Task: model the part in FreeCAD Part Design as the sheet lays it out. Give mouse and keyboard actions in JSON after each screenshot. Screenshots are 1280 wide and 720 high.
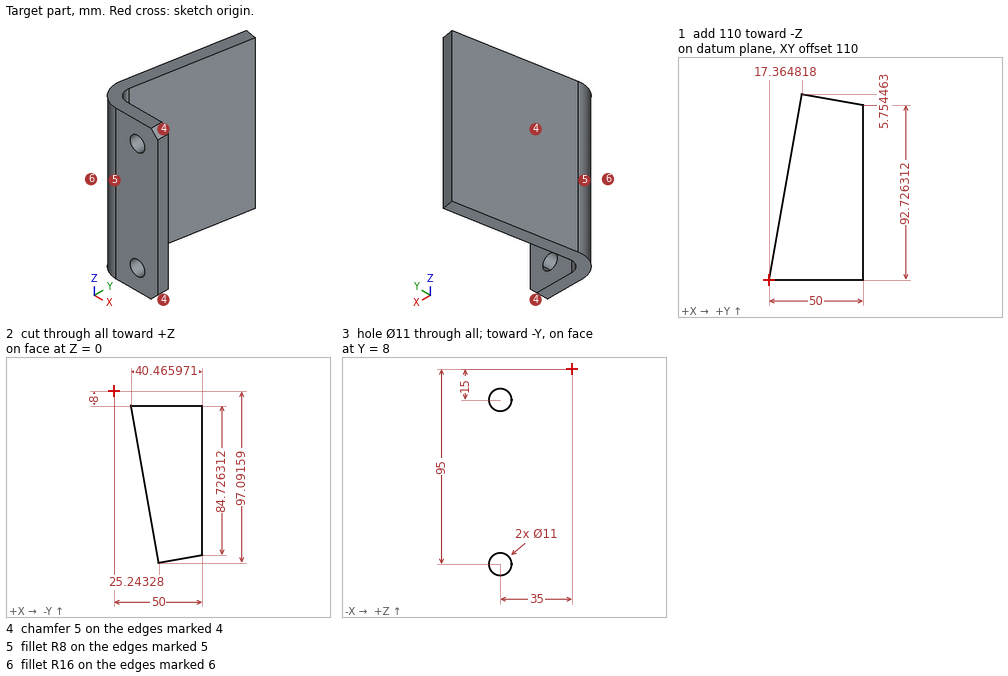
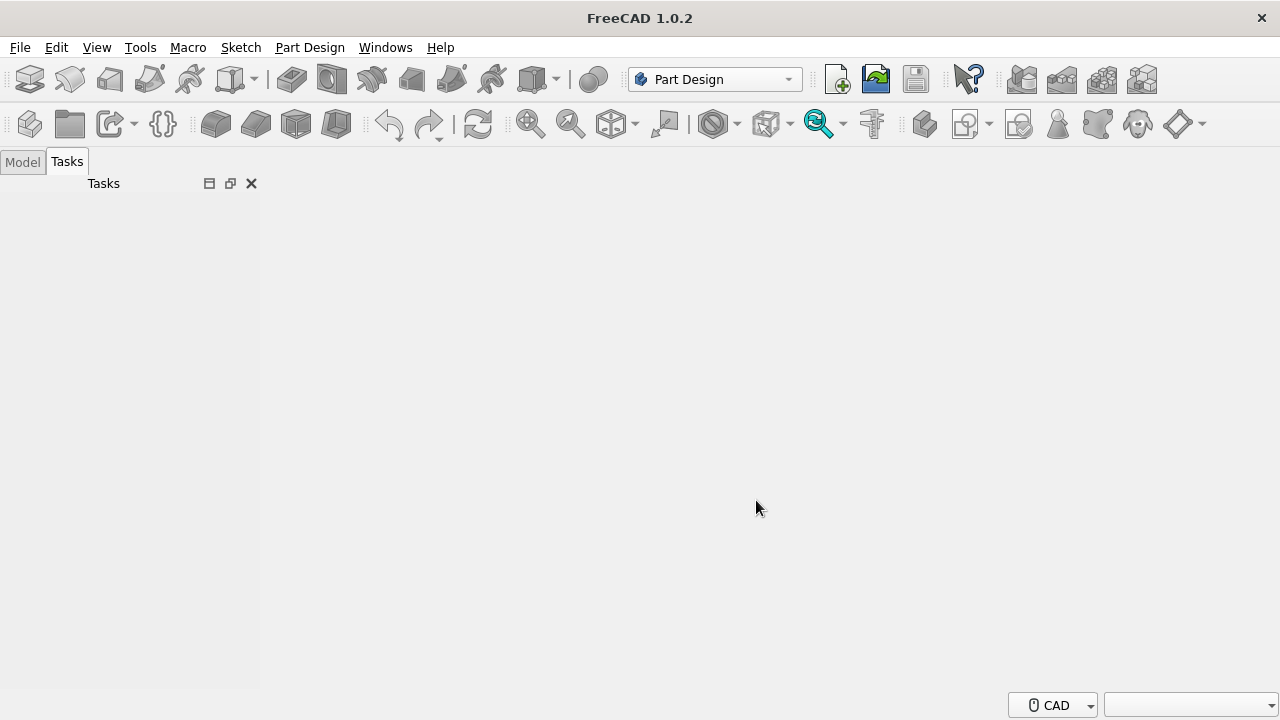
{"action": "left_click", "coordinate": [836, 80]}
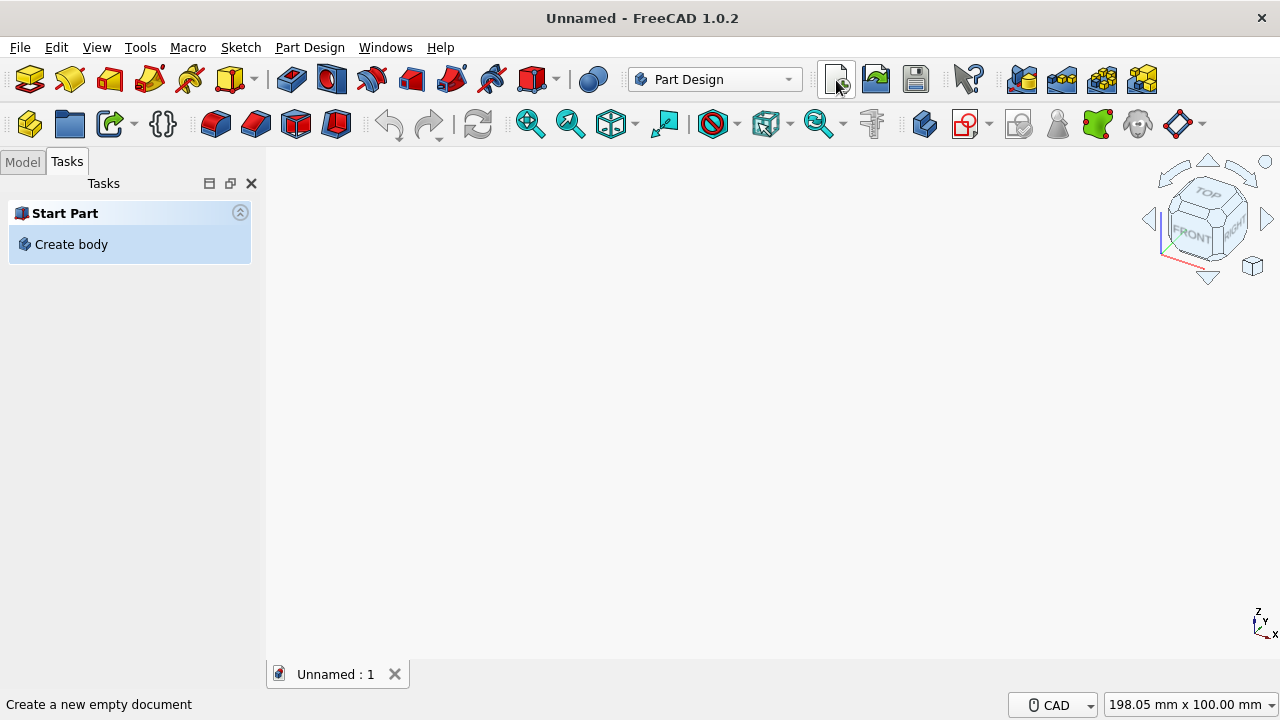
{"action": "left_click", "coordinate": [926, 124]}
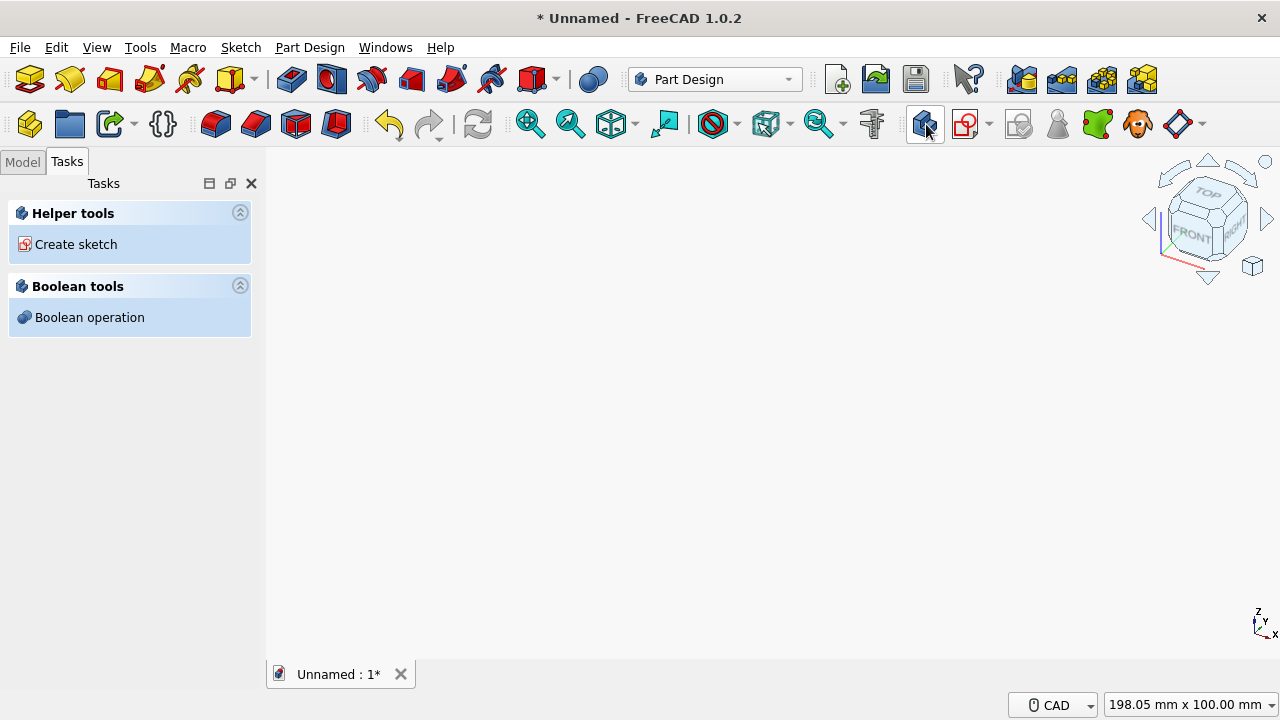
{"action": "left_click", "coordinate": [23, 161]}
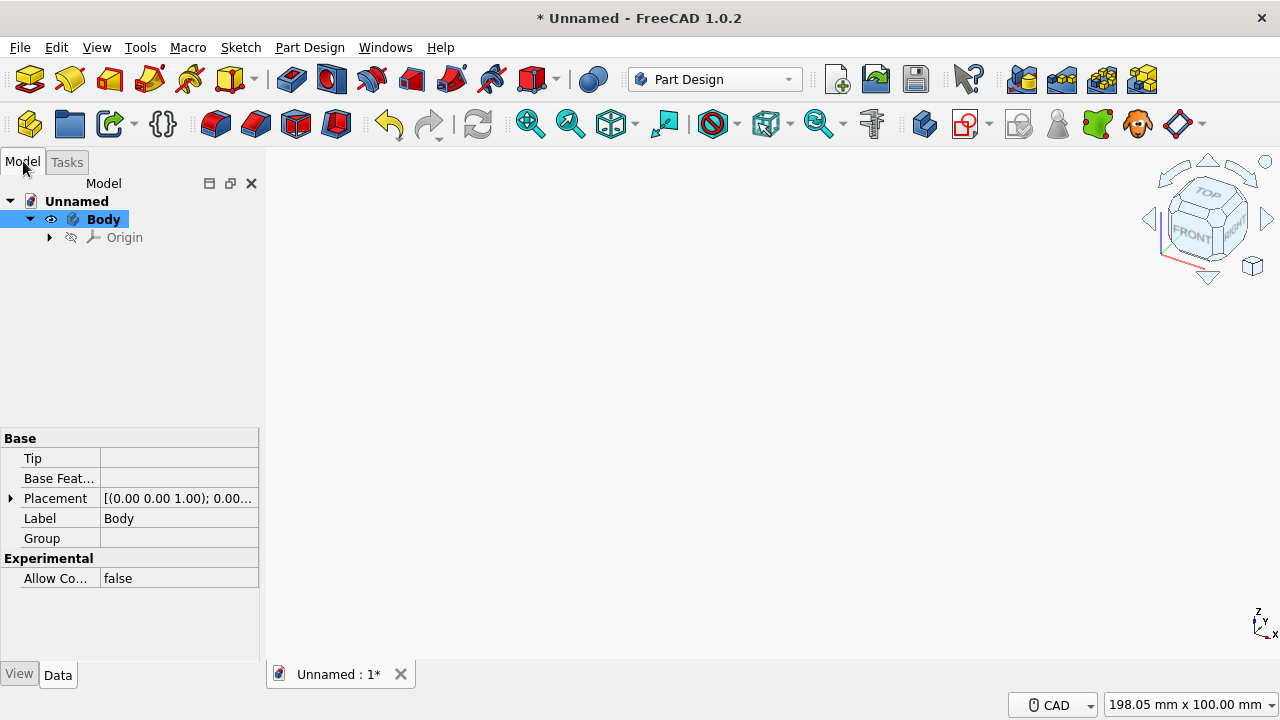
{"action": "left_click", "coordinate": [50, 237]}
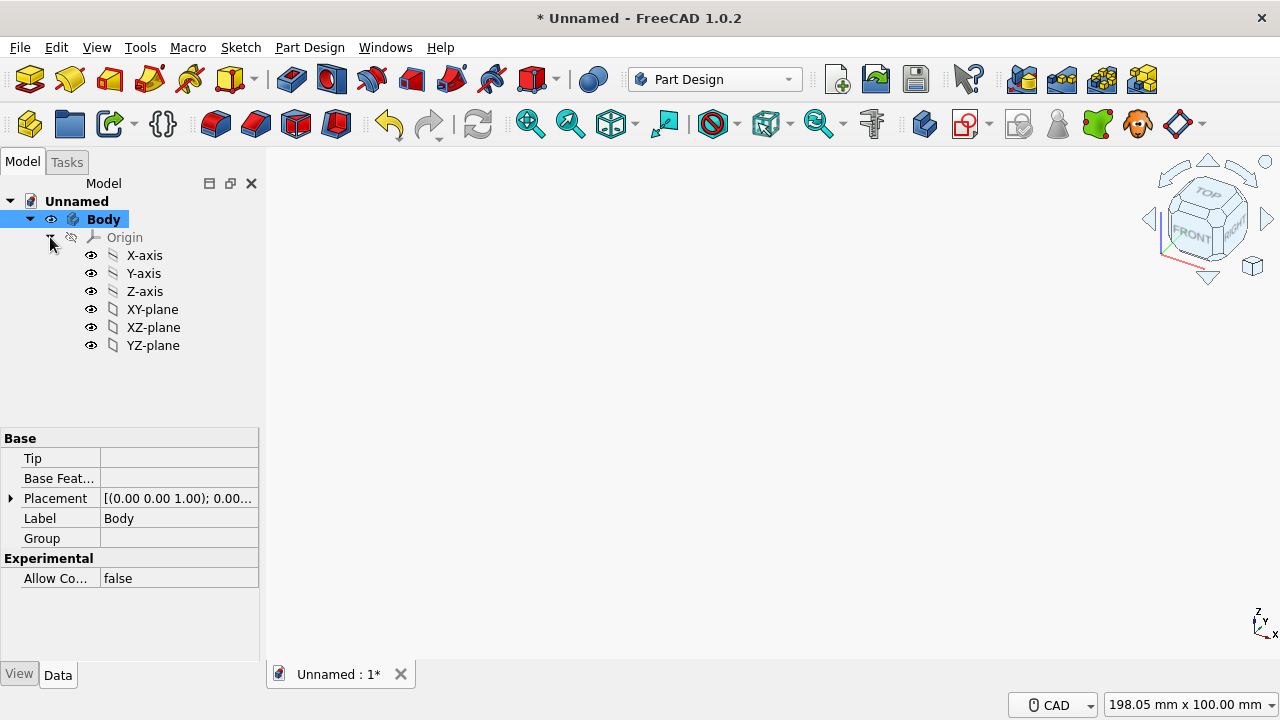
{"action": "left_click", "coordinate": [136, 309]}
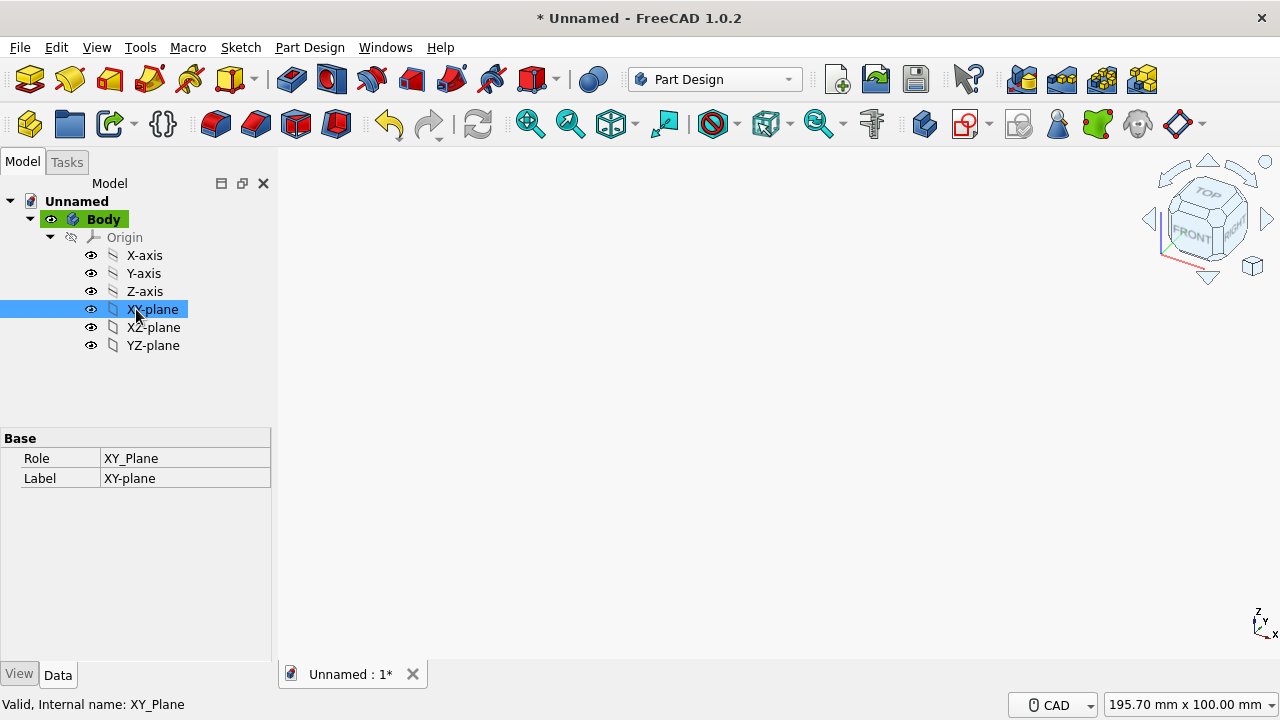
{"action": "left_click", "coordinate": [1178, 124]}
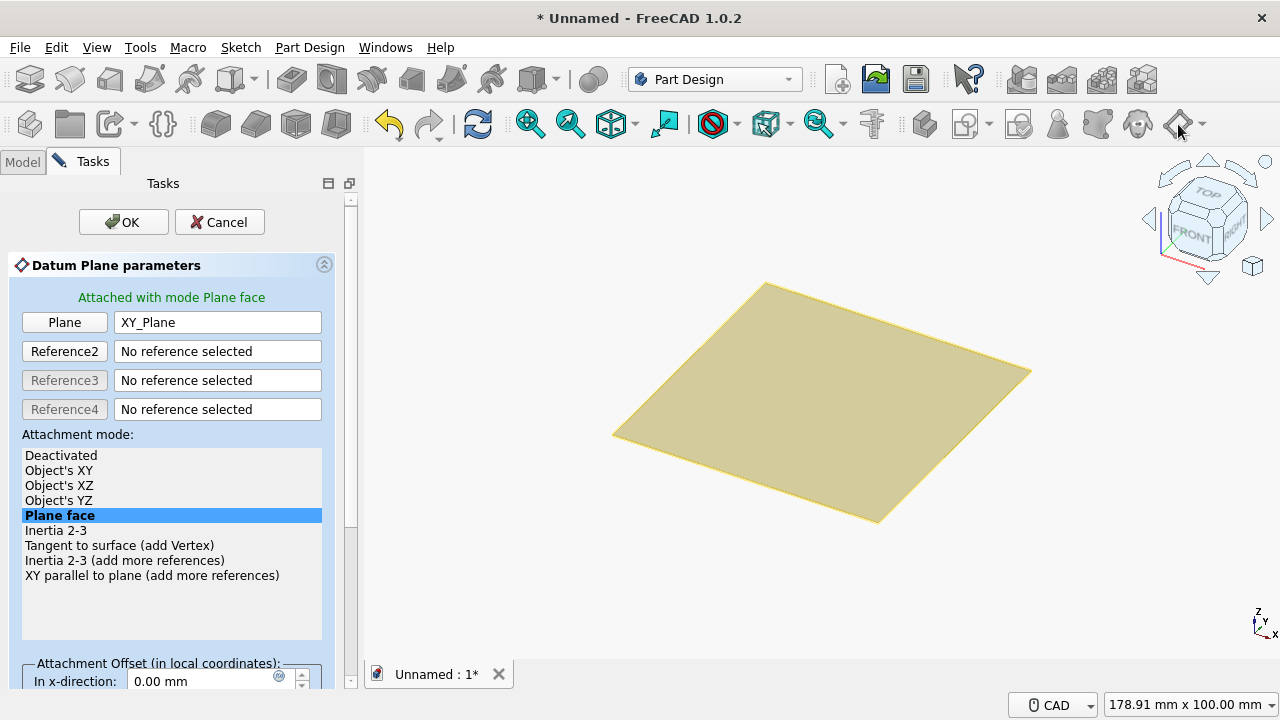
{"action": "scroll", "coordinate": [351, 440], "scroll_direction": "down", "scroll_amount": 3}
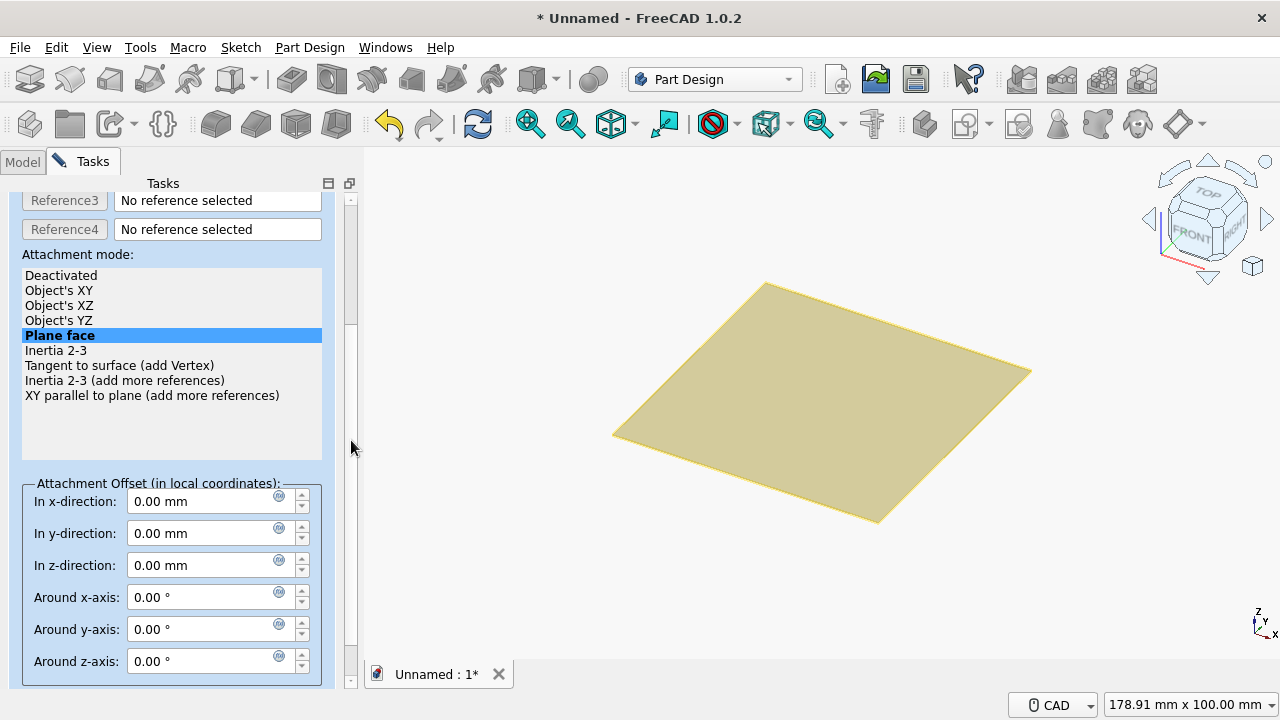
{"action": "triple_click", "coordinate": [210, 565]}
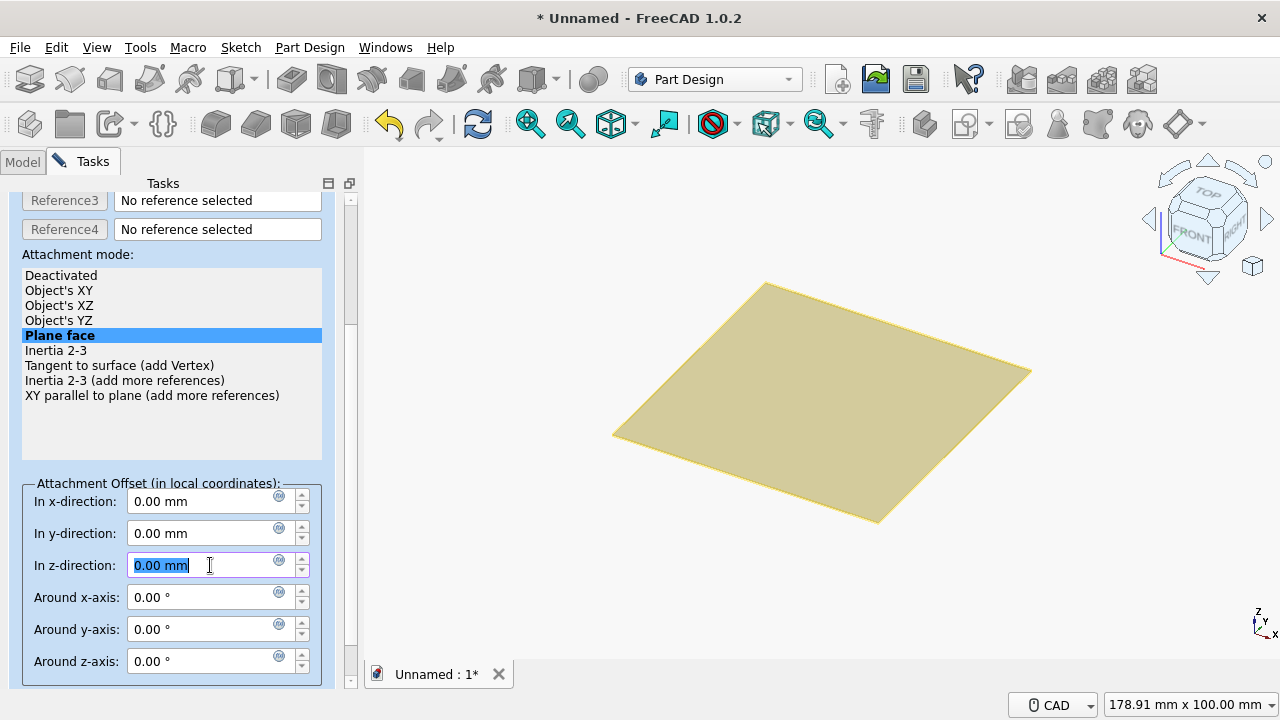
{"action": "type", "text": "110"}
{"action": "key", "text": "Tab"}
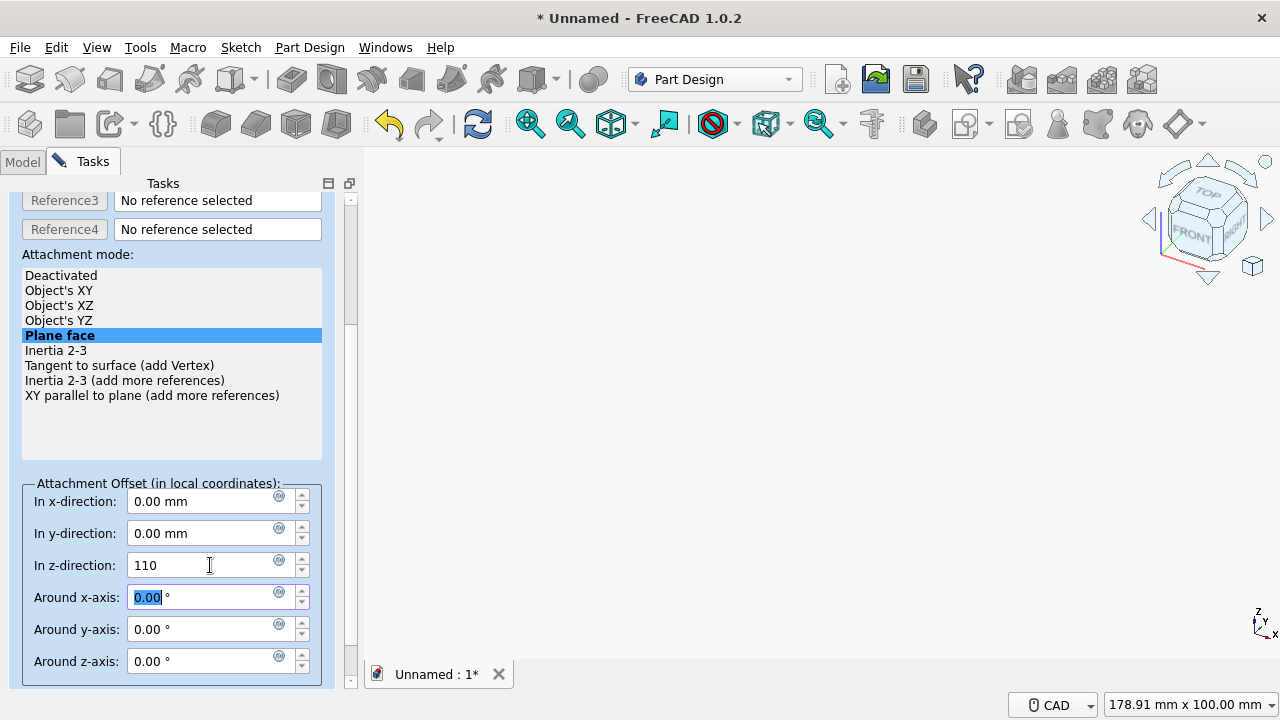
{"action": "scroll", "coordinate": [351, 440], "scroll_direction": "up", "scroll_amount": 4}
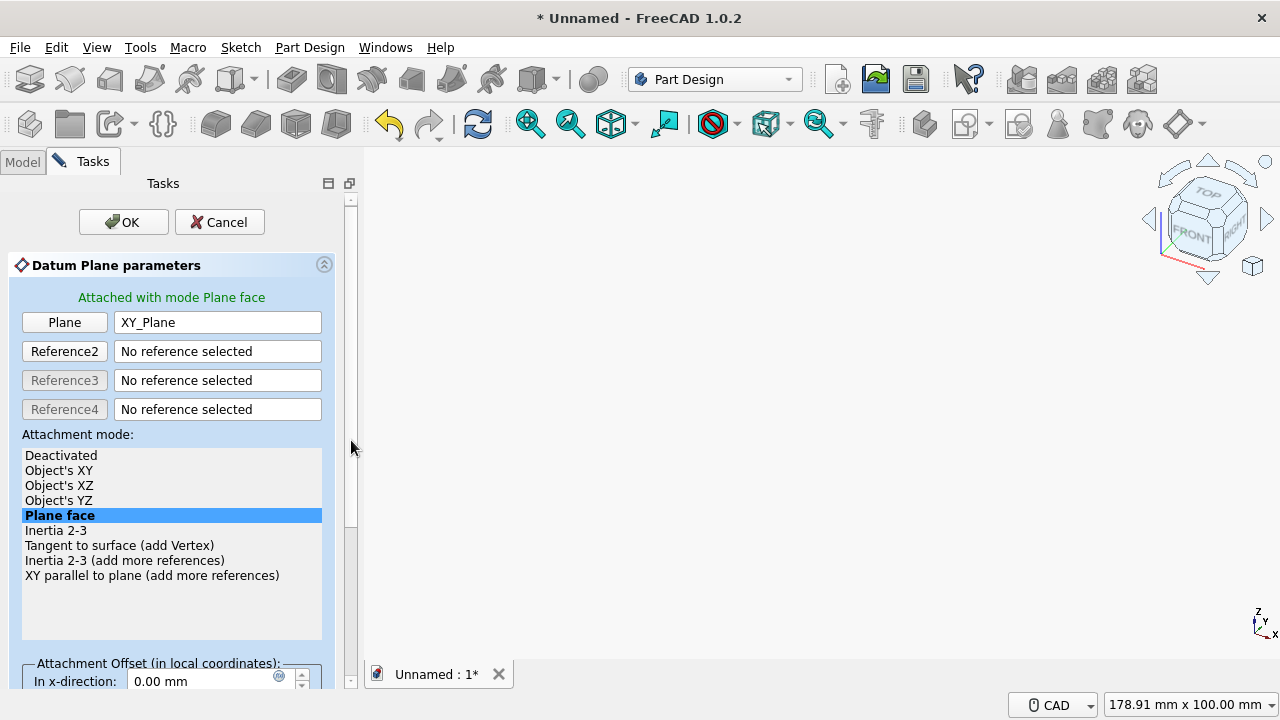
{"action": "left_click", "coordinate": [124, 222]}